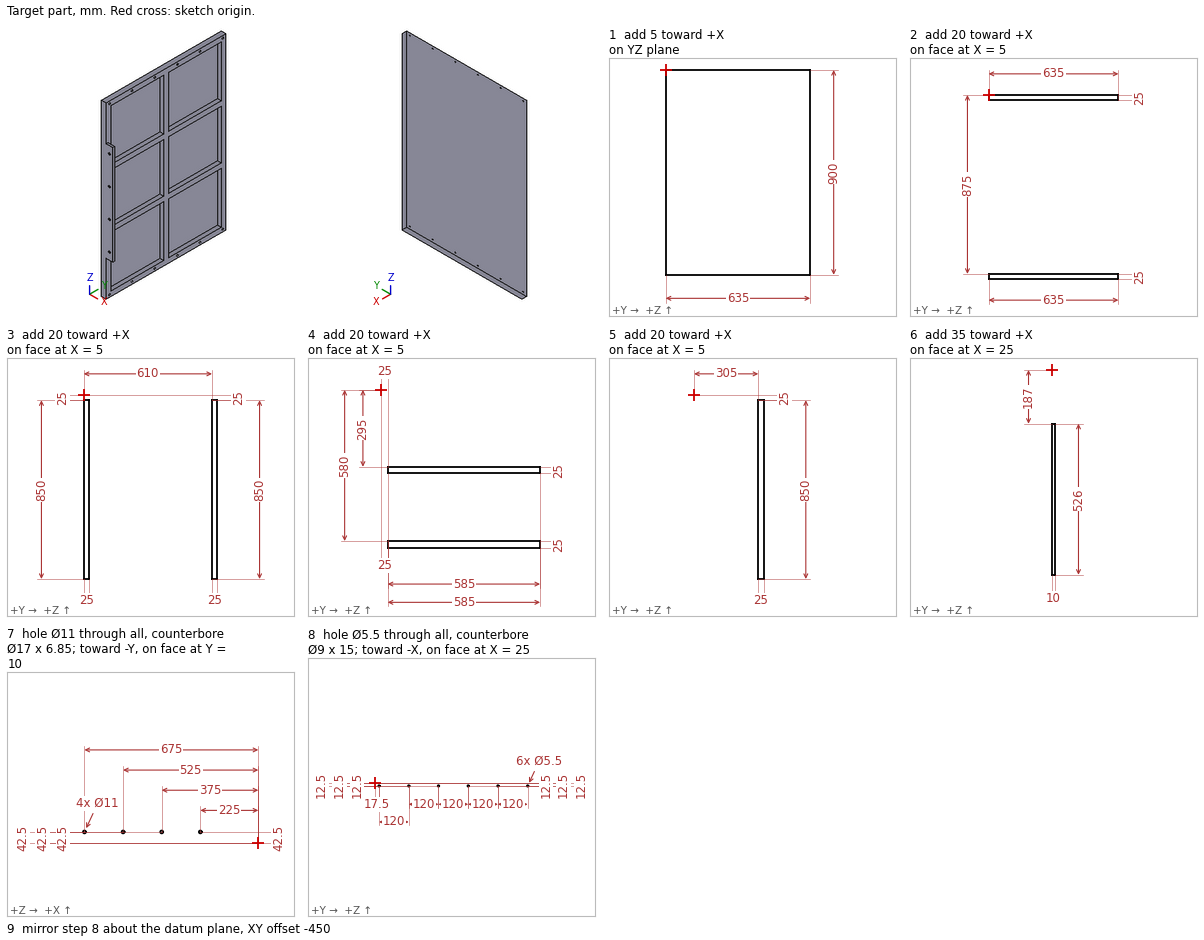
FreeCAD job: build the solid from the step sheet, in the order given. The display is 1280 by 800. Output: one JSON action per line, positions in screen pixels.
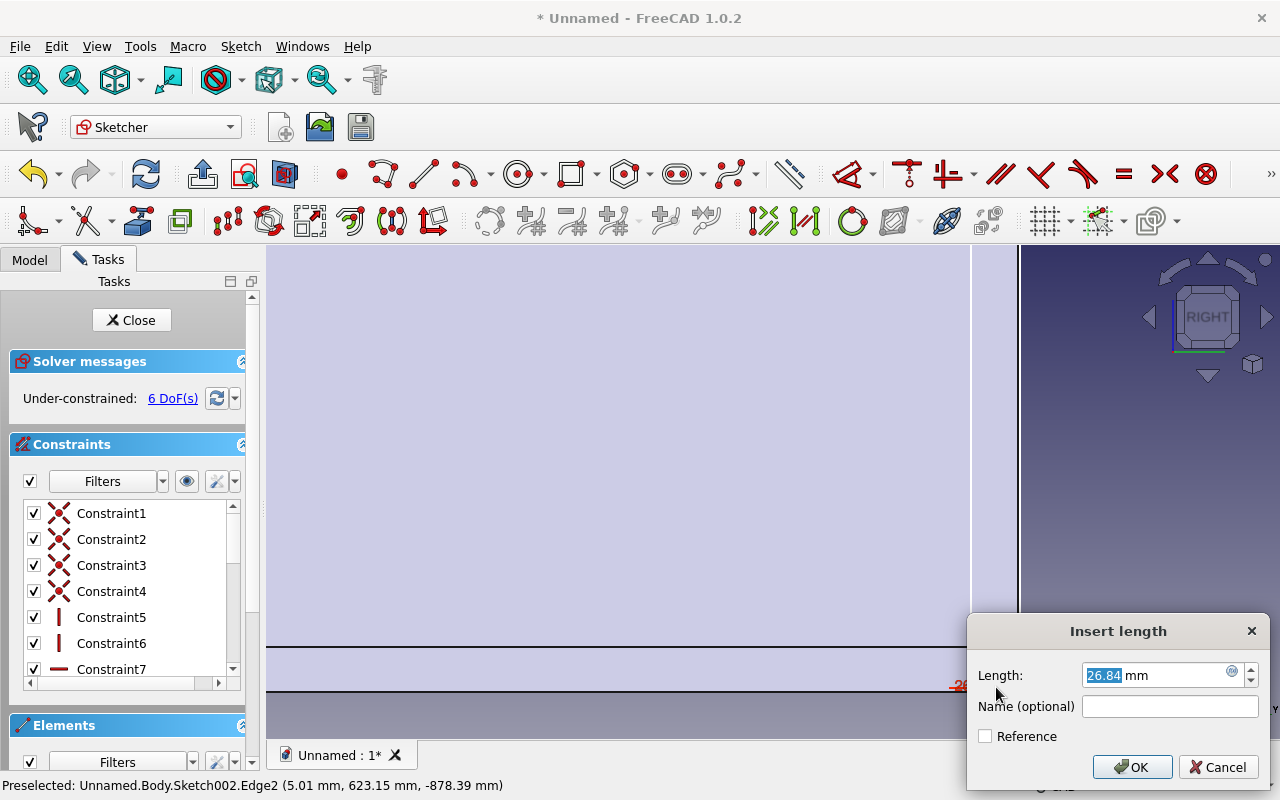
{"action": "type", "text": "25"}
{"action": "key", "text": "Return"}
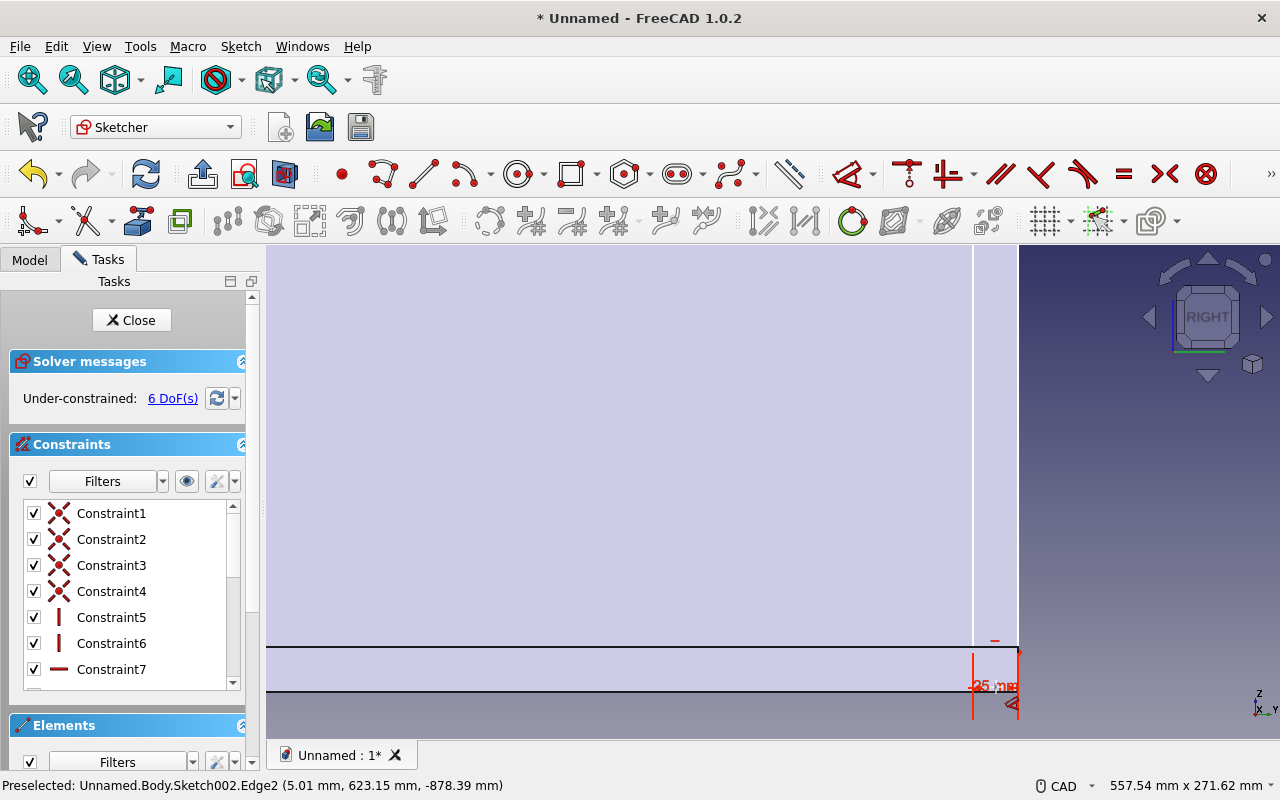
{"action": "scroll", "coordinate": [771, 654], "scroll_direction": "down", "scroll_amount": 8}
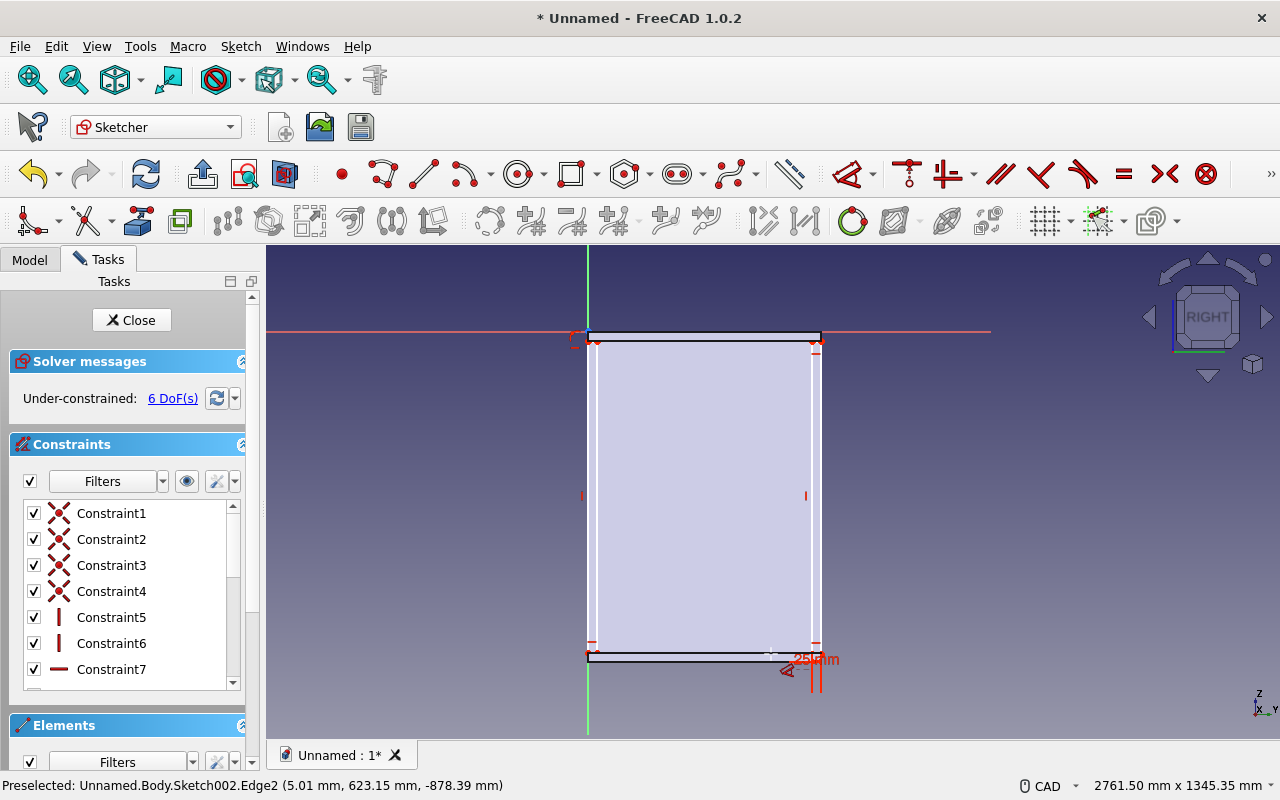
{"action": "scroll", "coordinate": [591, 654], "scroll_direction": "up", "scroll_amount": 9}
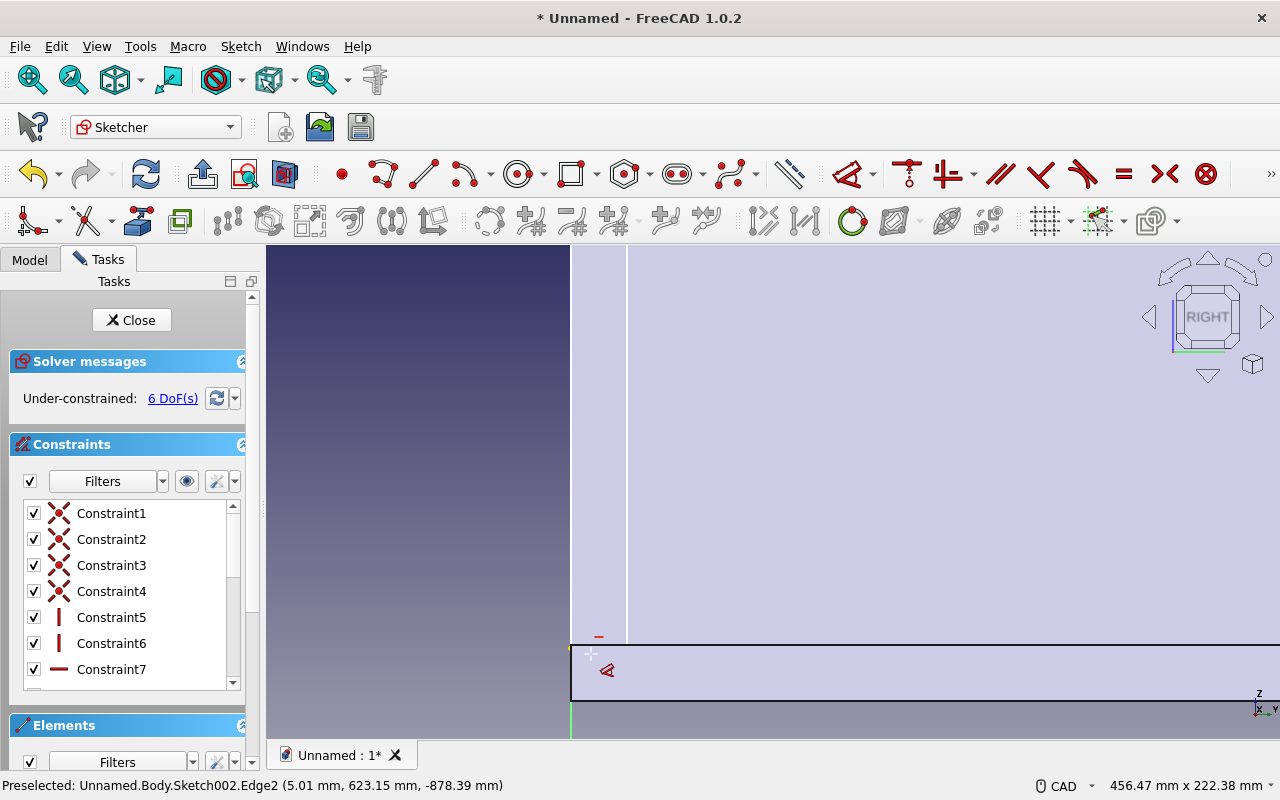
{"action": "left_click", "coordinate": [588, 649]}
{"action": "left_click", "coordinate": [599, 683]}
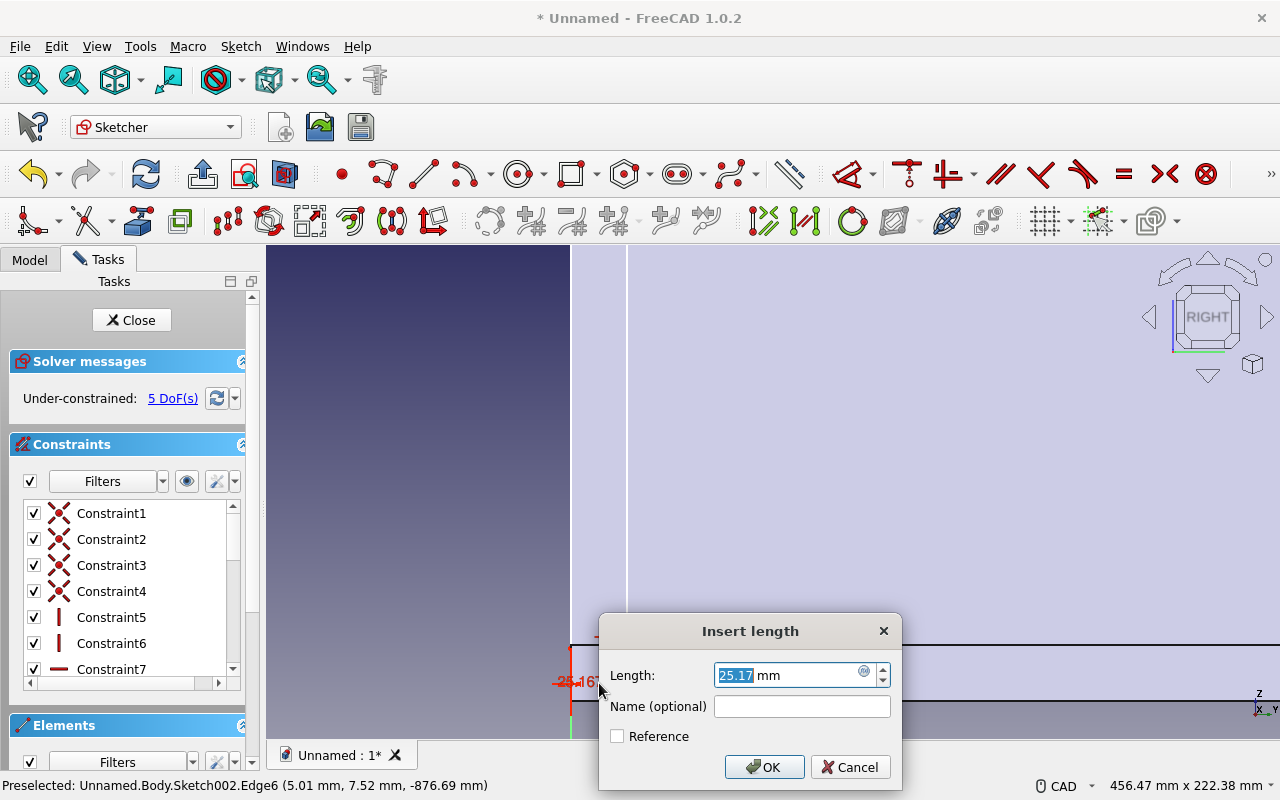
{"action": "type", "text": "25"}
{"action": "key", "text": "Return"}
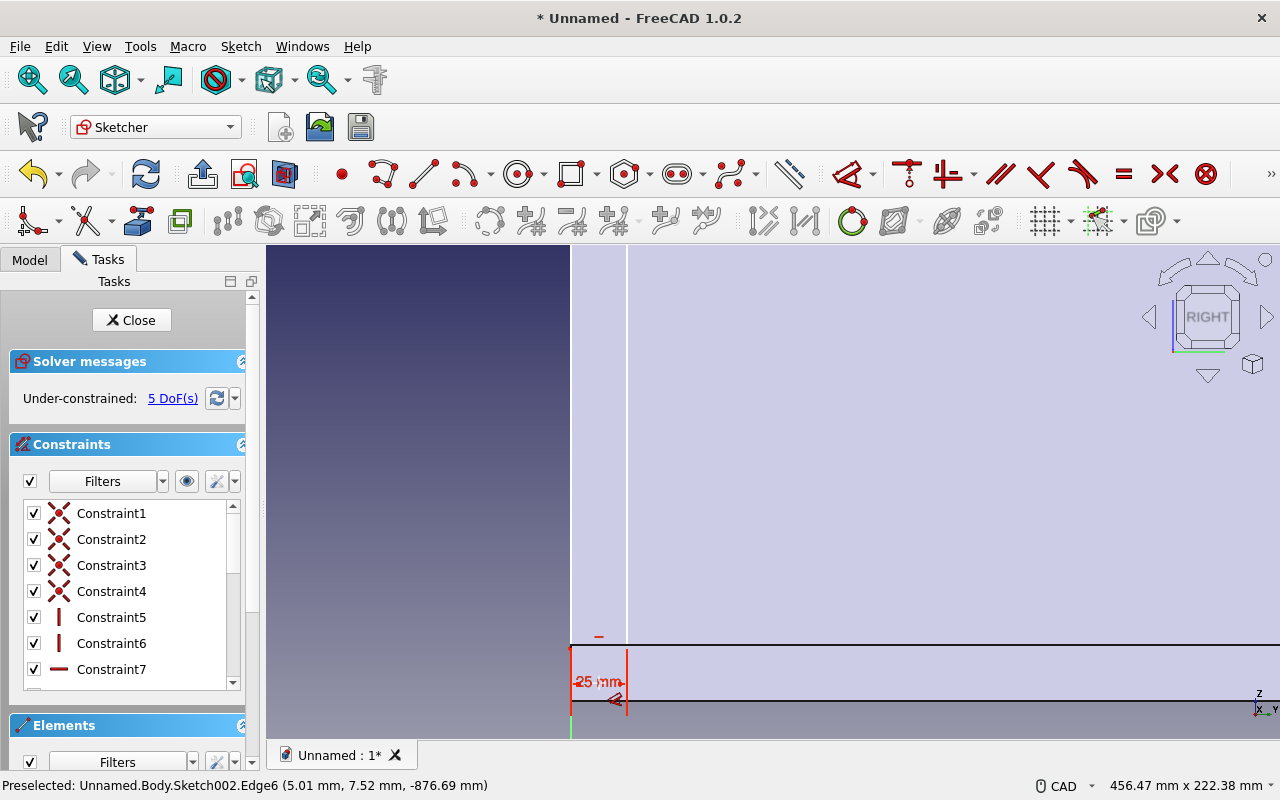
{"action": "scroll", "coordinate": [591, 654], "scroll_direction": "down", "scroll_amount": 9}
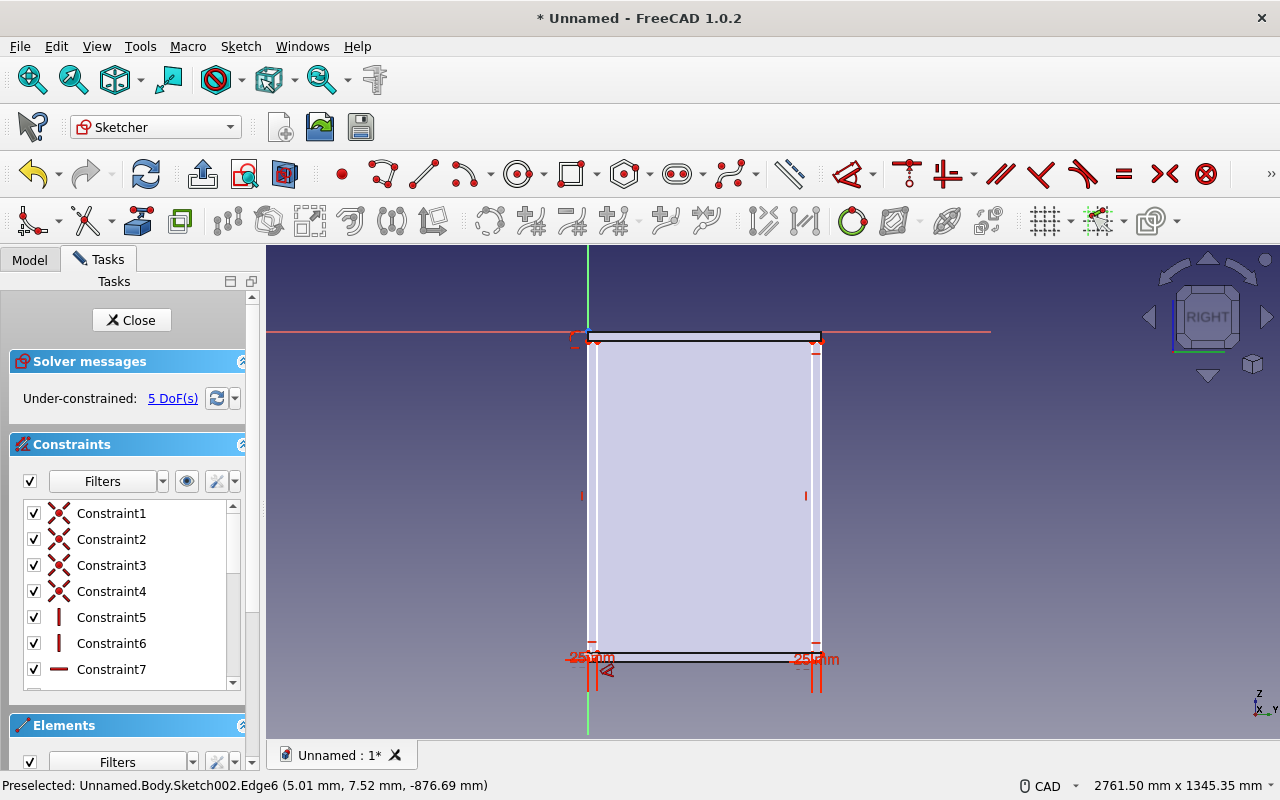
{"action": "scroll", "coordinate": [812, 435], "scroll_direction": "up", "scroll_amount": 3}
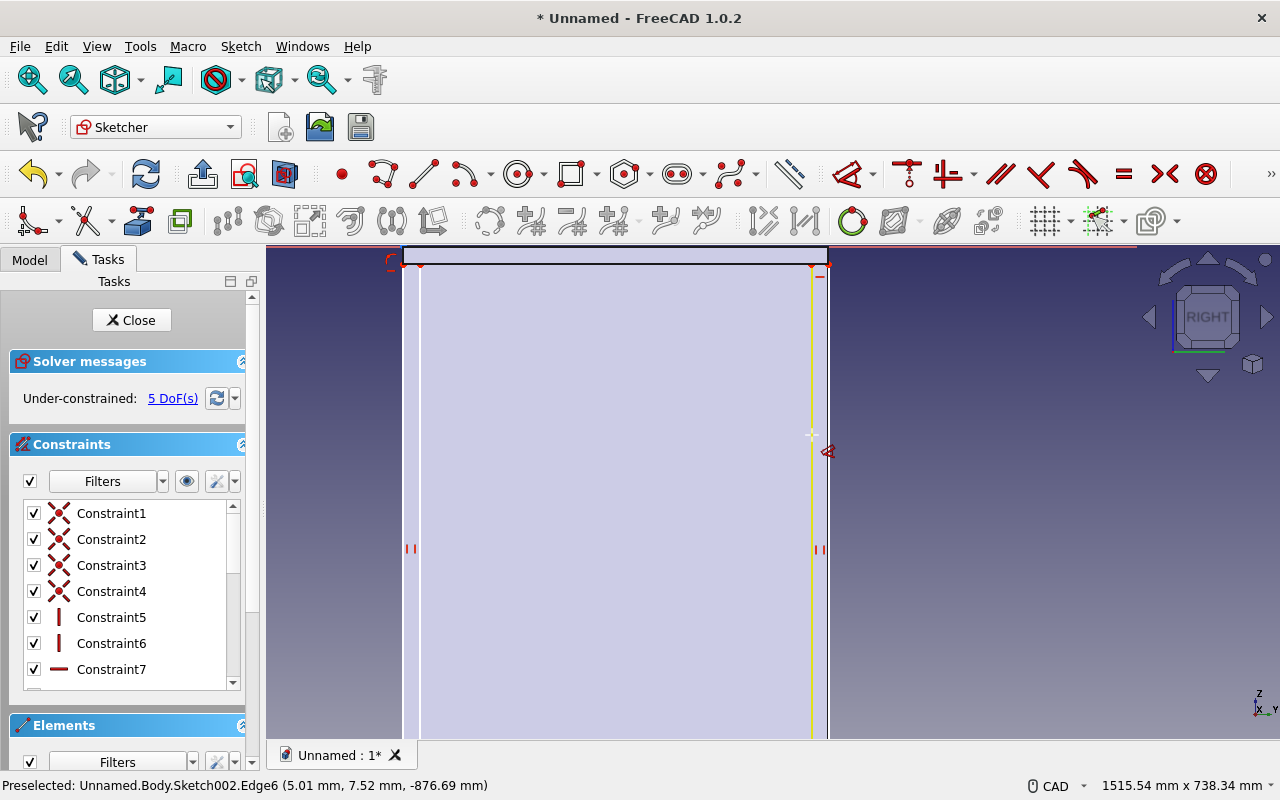
{"action": "left_click", "coordinate": [812, 435]}
{"action": "left_click", "coordinate": [846, 492]}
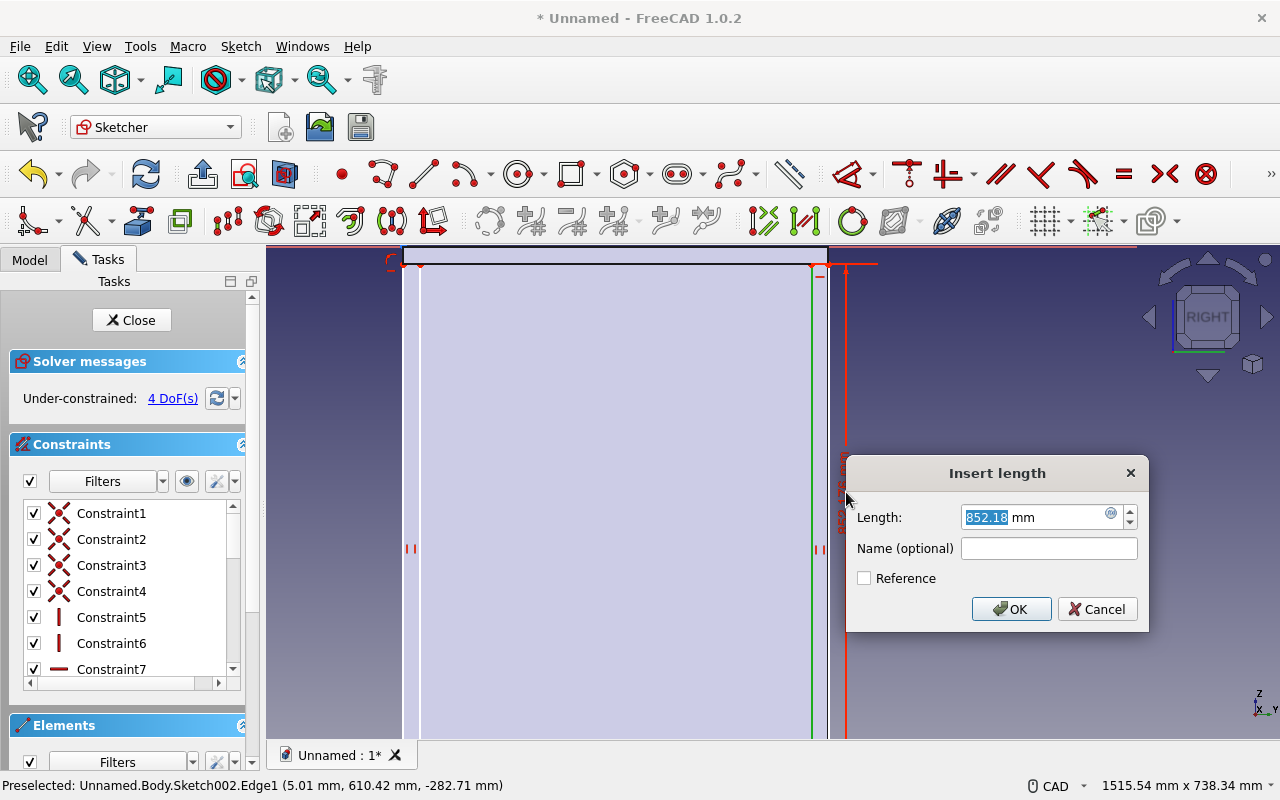
{"action": "type", "text": "850"}
{"action": "key", "text": "Return"}